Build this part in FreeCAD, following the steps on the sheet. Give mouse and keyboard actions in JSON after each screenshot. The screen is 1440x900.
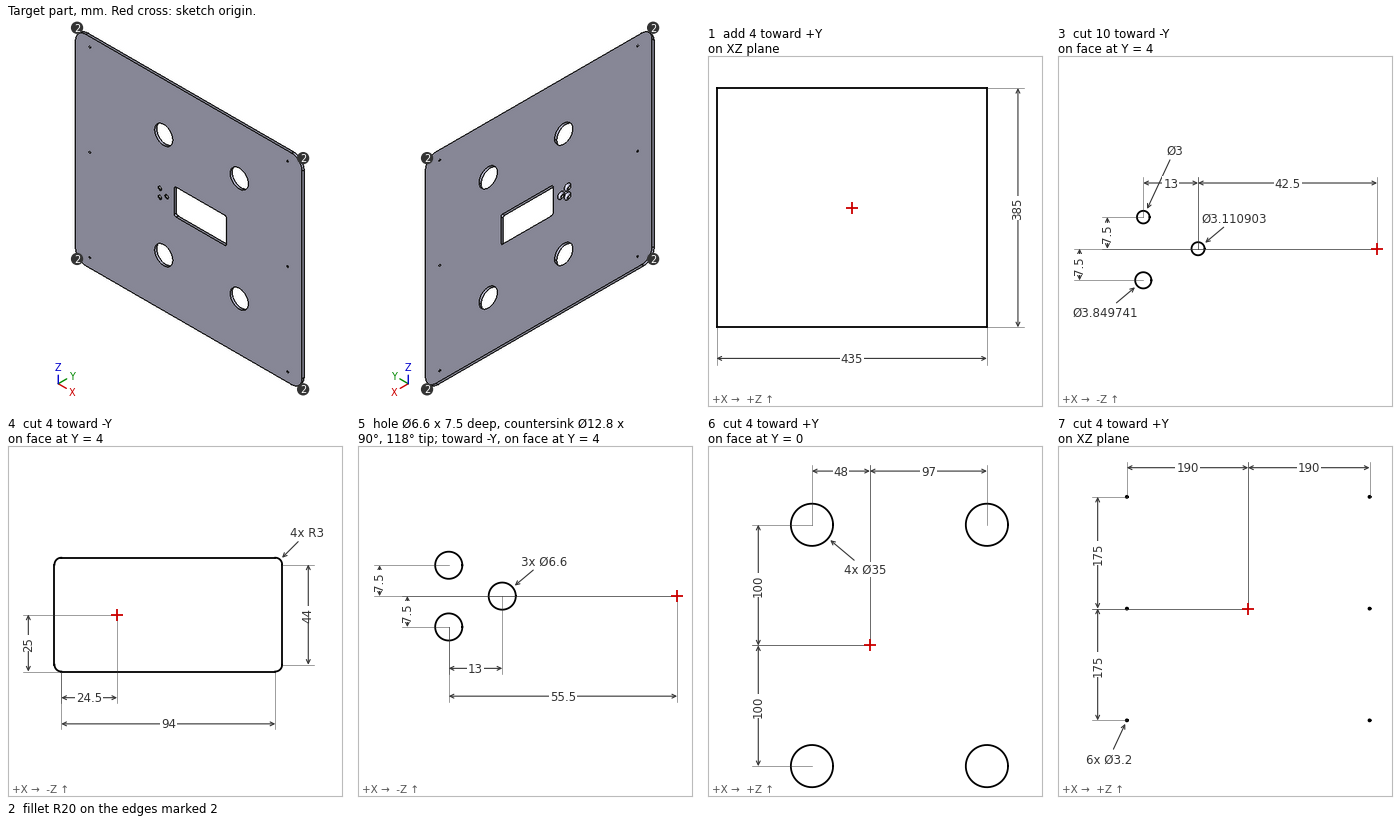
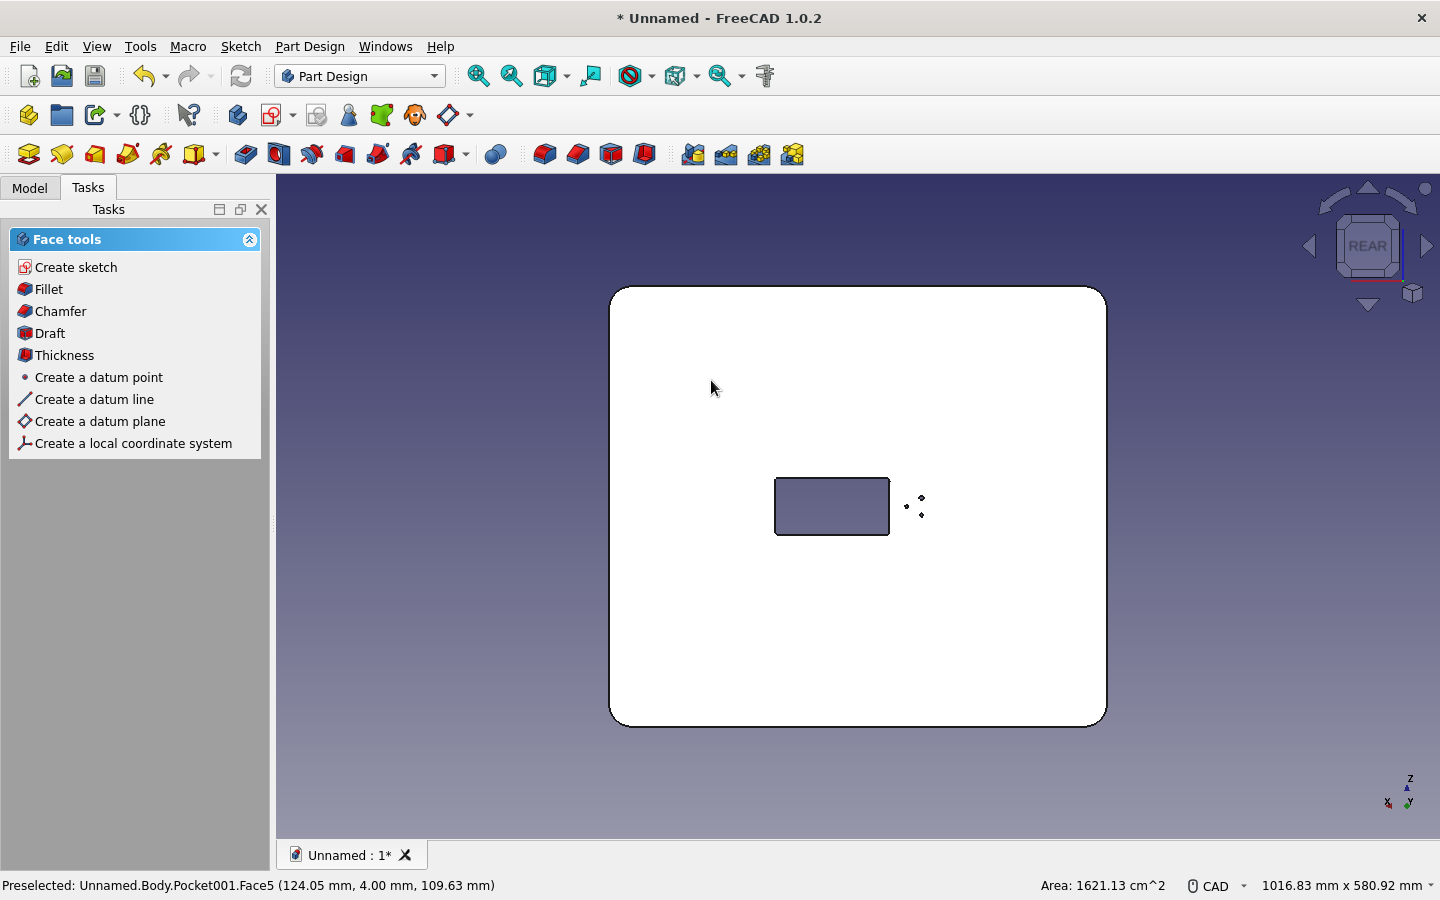
{"action": "left_click", "coordinate": [270, 116]}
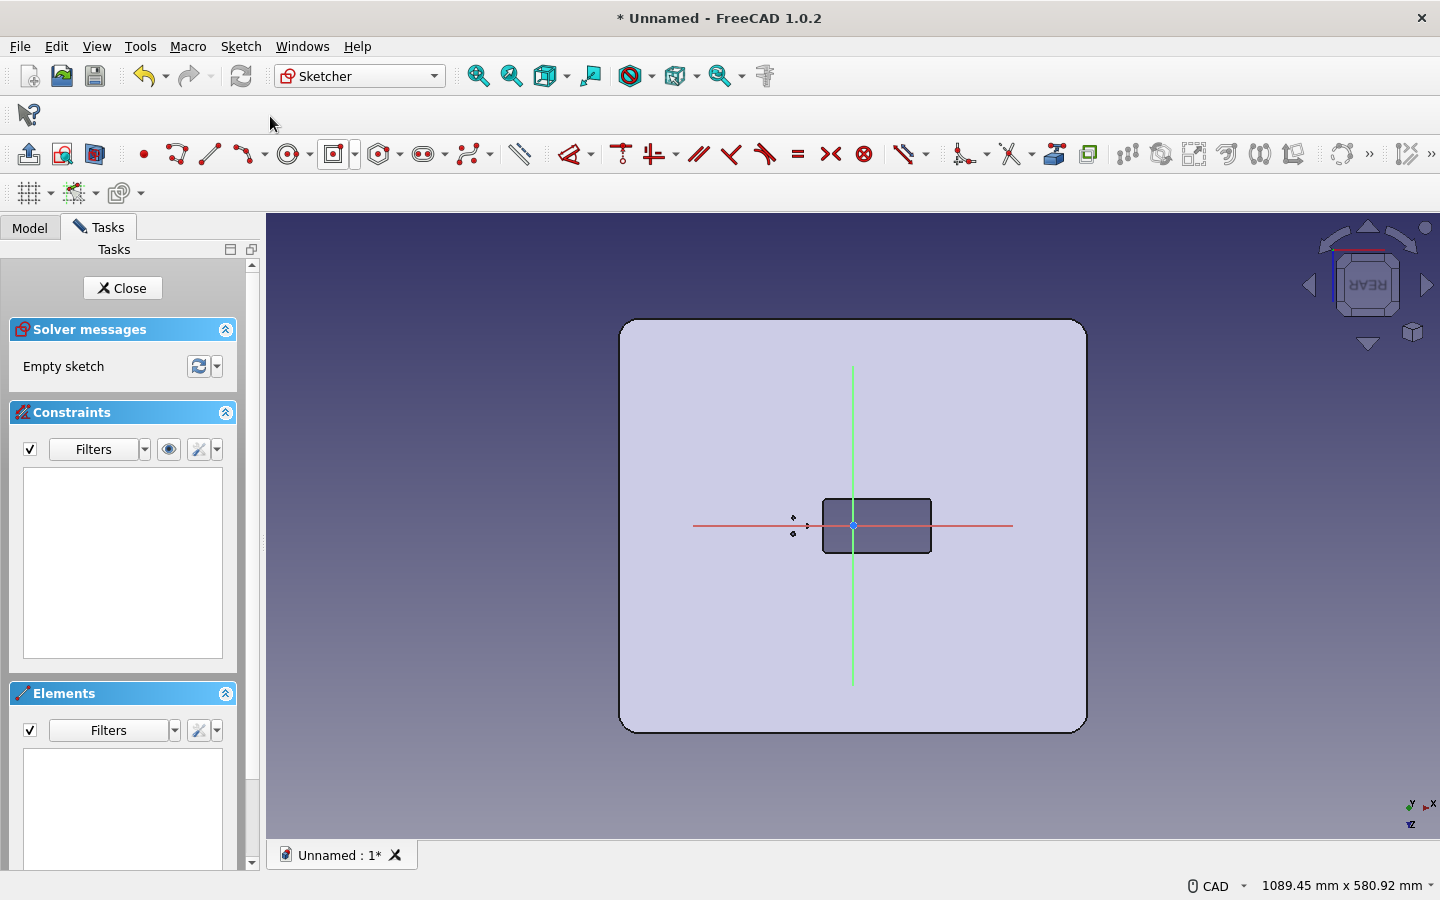
{"action": "scroll", "coordinate": [801, 526], "scroll_direction": "up", "scroll_amount": 14}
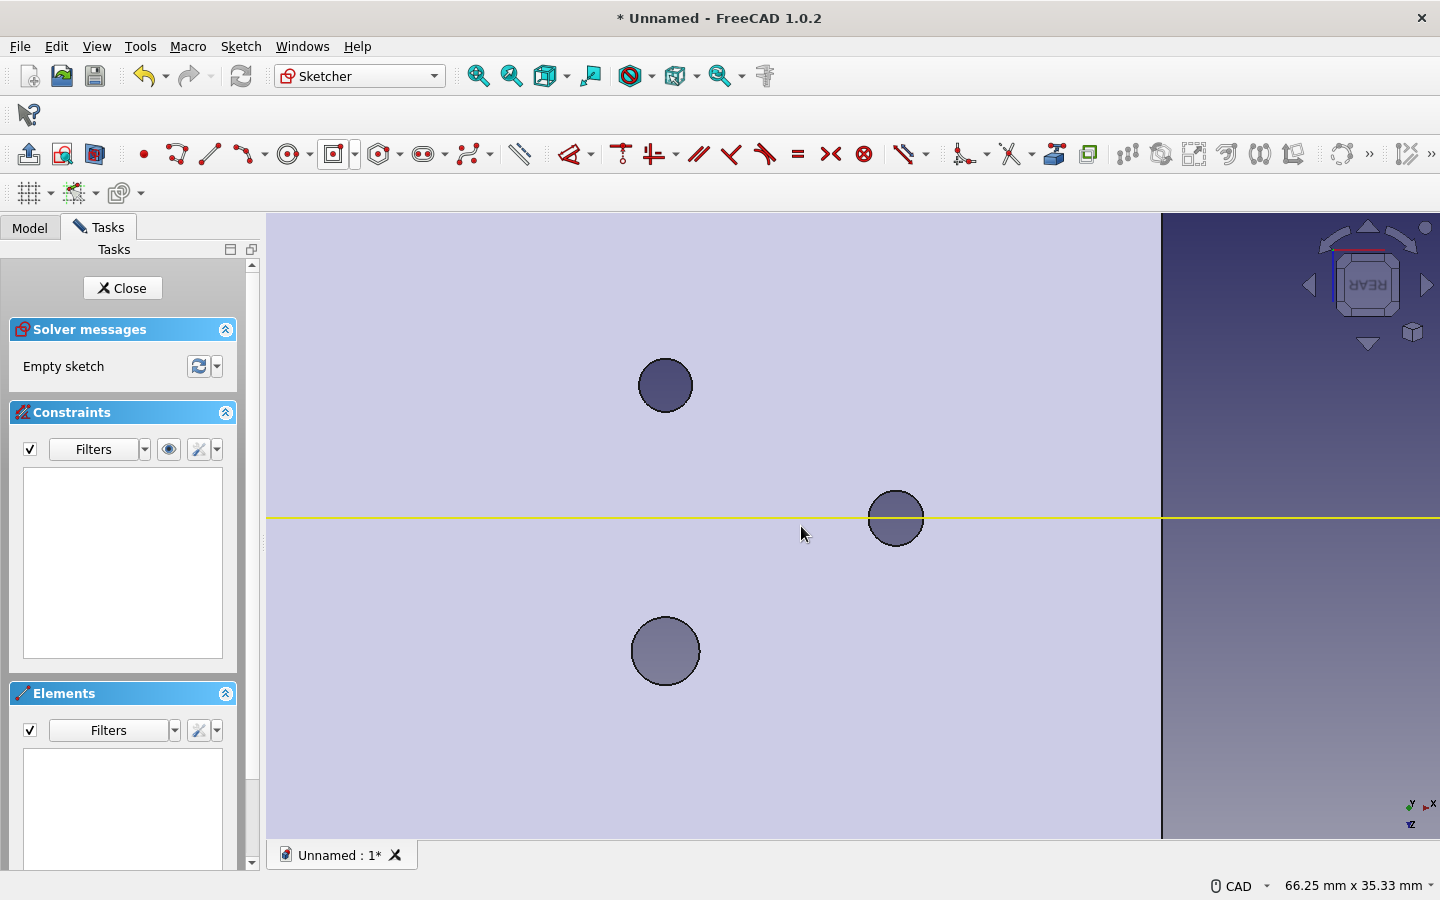
{"action": "left_click", "coordinate": [288, 154]}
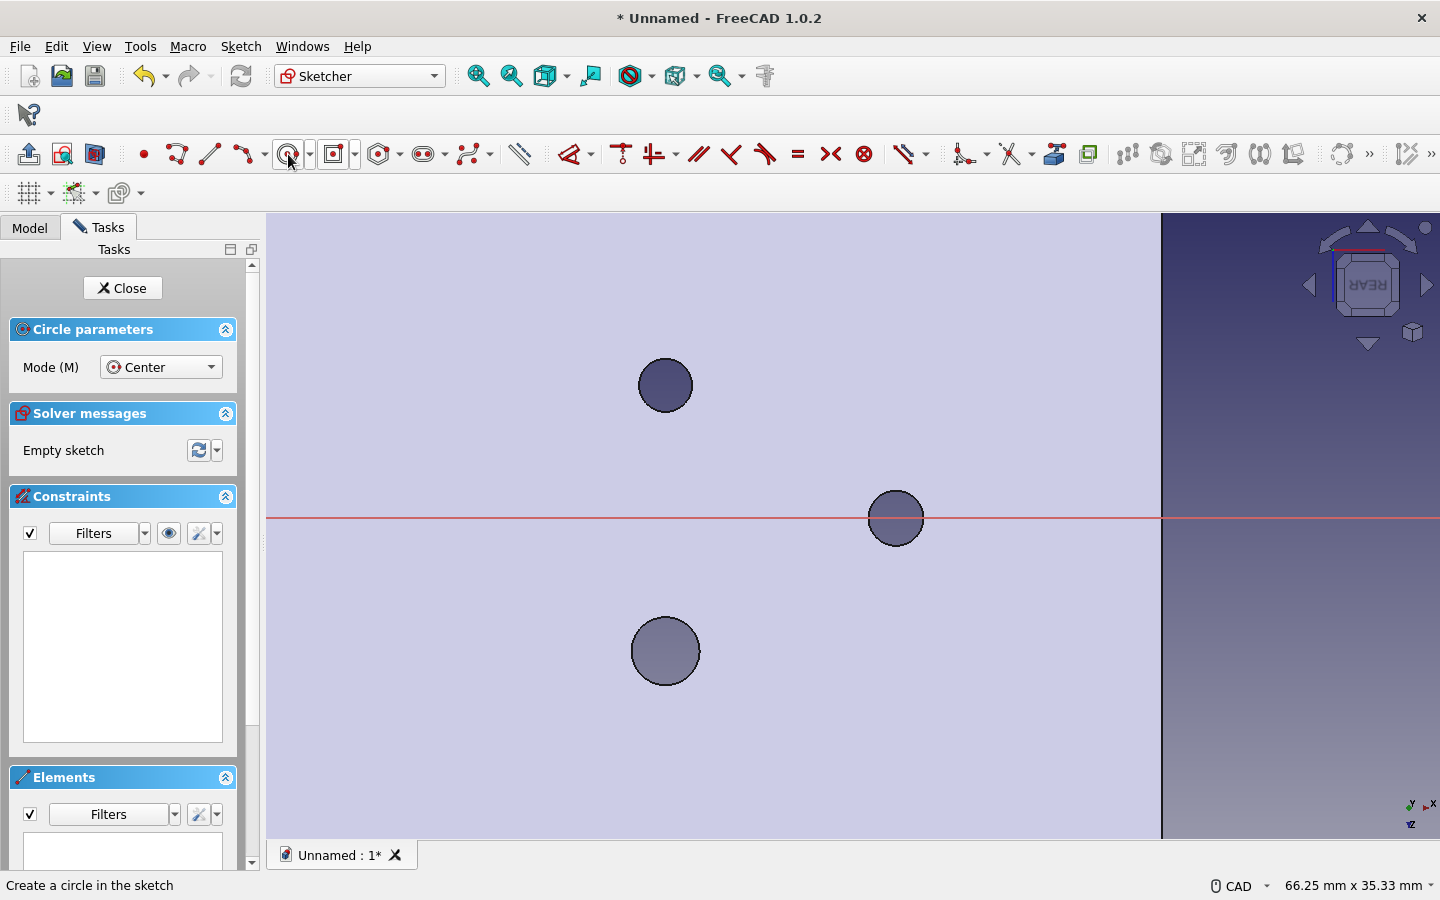
{"action": "left_click", "coordinate": [666, 651]}
{"action": "left_click", "coordinate": [707, 610]}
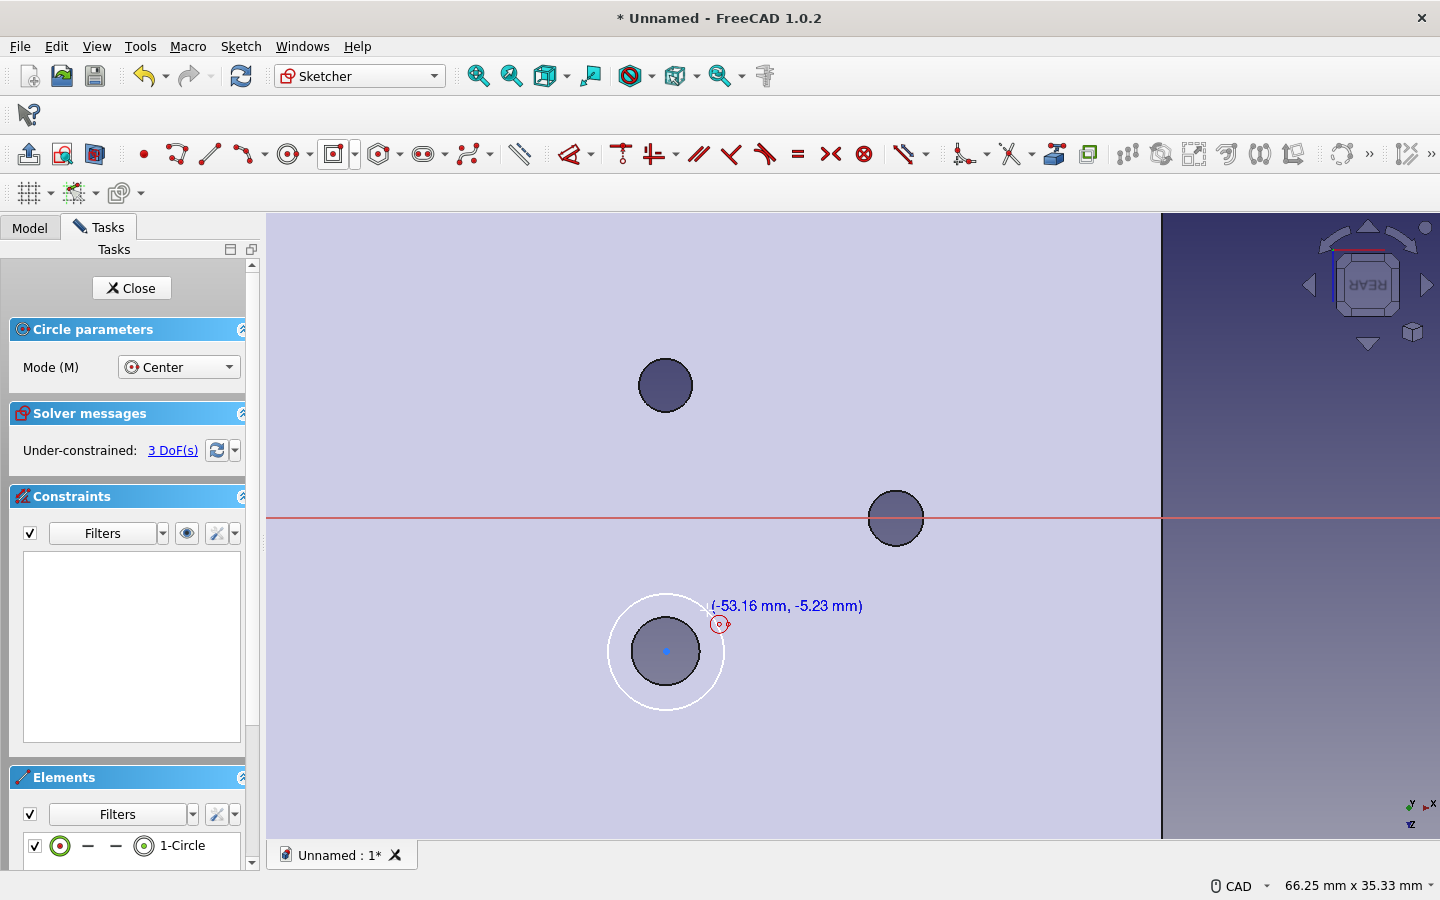
{"action": "left_click", "coordinate": [896, 518]}
{"action": "left_click", "coordinate": [937, 477]}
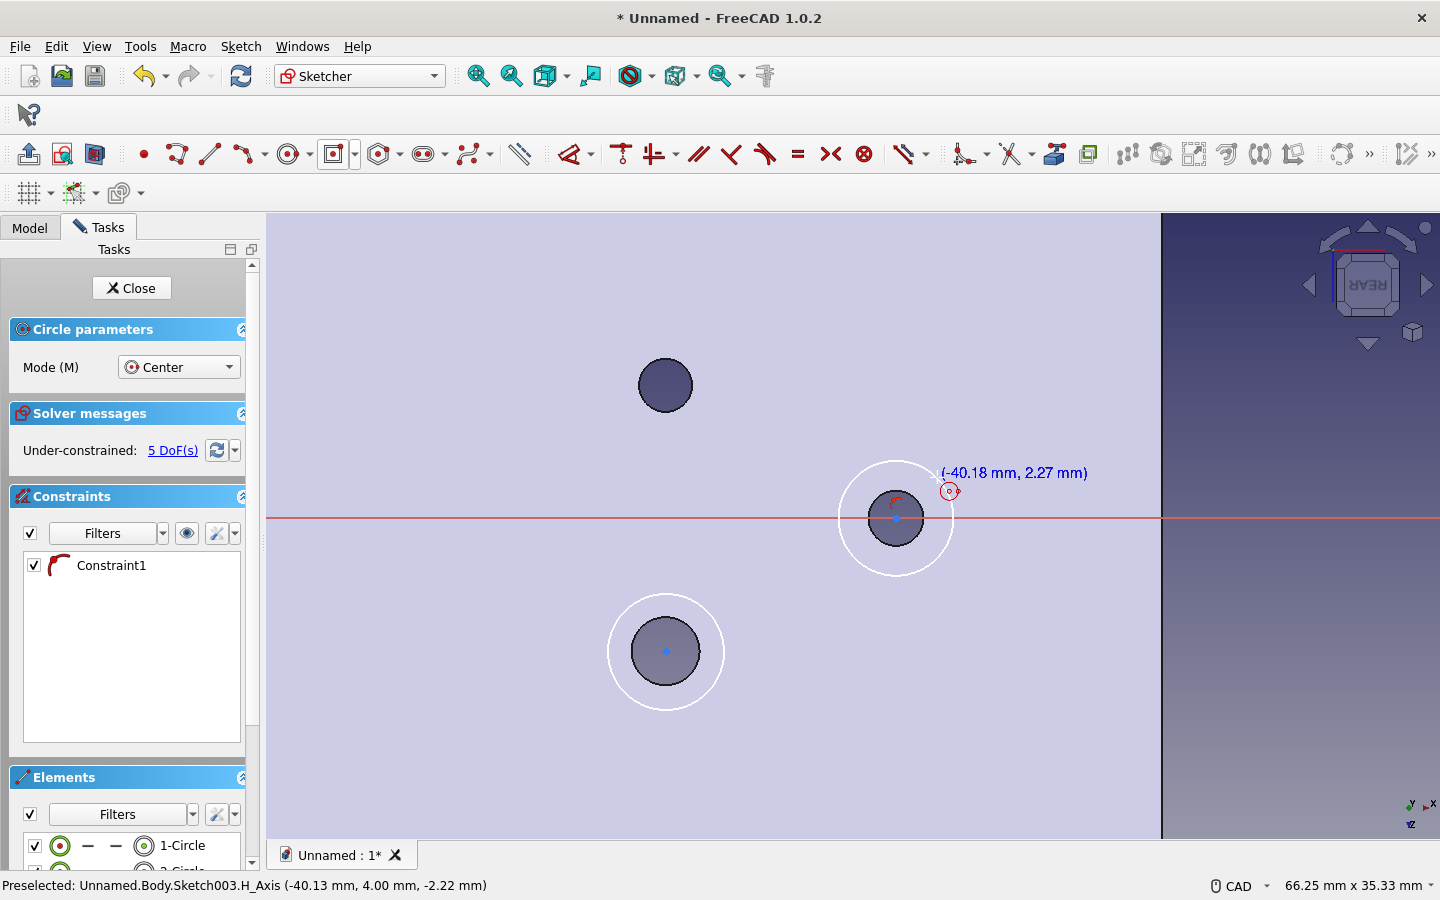
{"action": "left_click", "coordinate": [666, 385]}
{"action": "left_click", "coordinate": [707, 344]}
{"action": "key", "text": "Escape"}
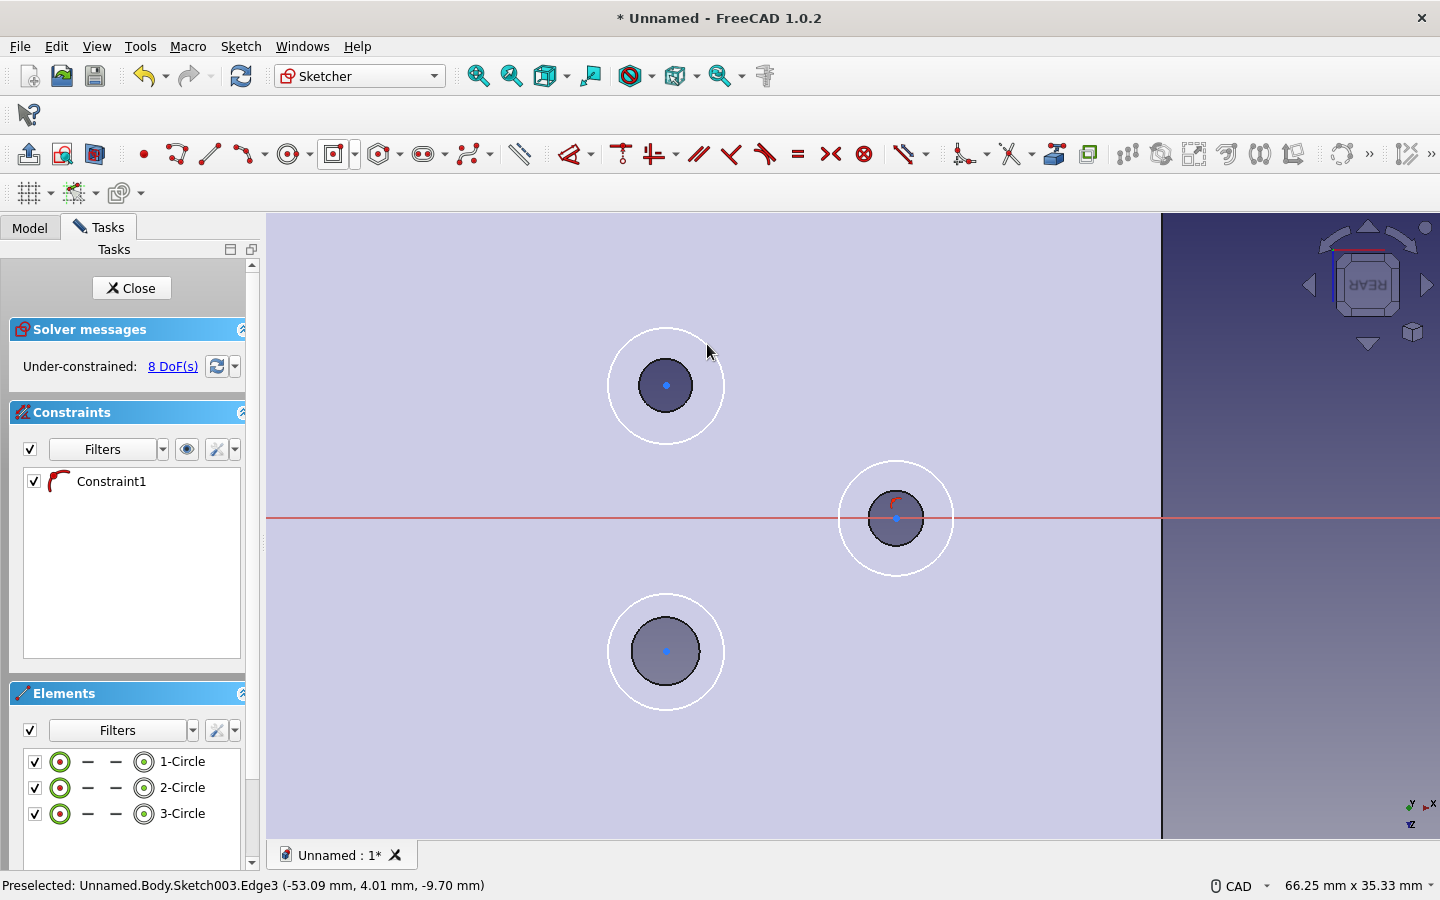
{"action": "left_click", "coordinate": [707, 611]}